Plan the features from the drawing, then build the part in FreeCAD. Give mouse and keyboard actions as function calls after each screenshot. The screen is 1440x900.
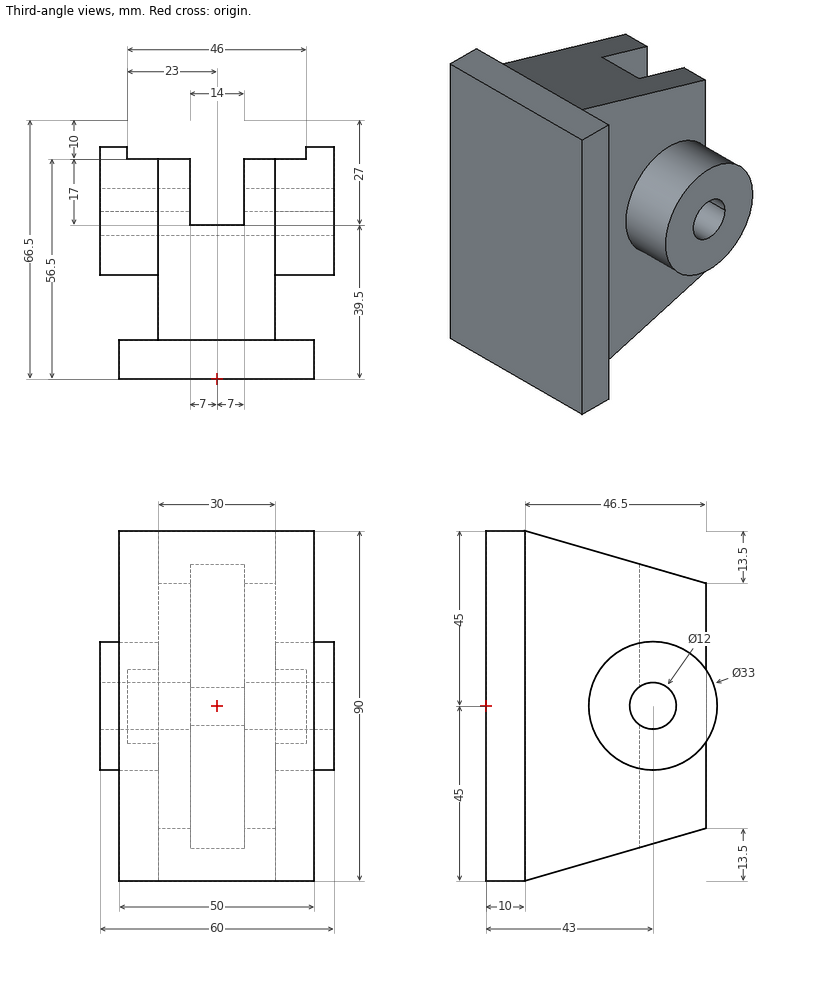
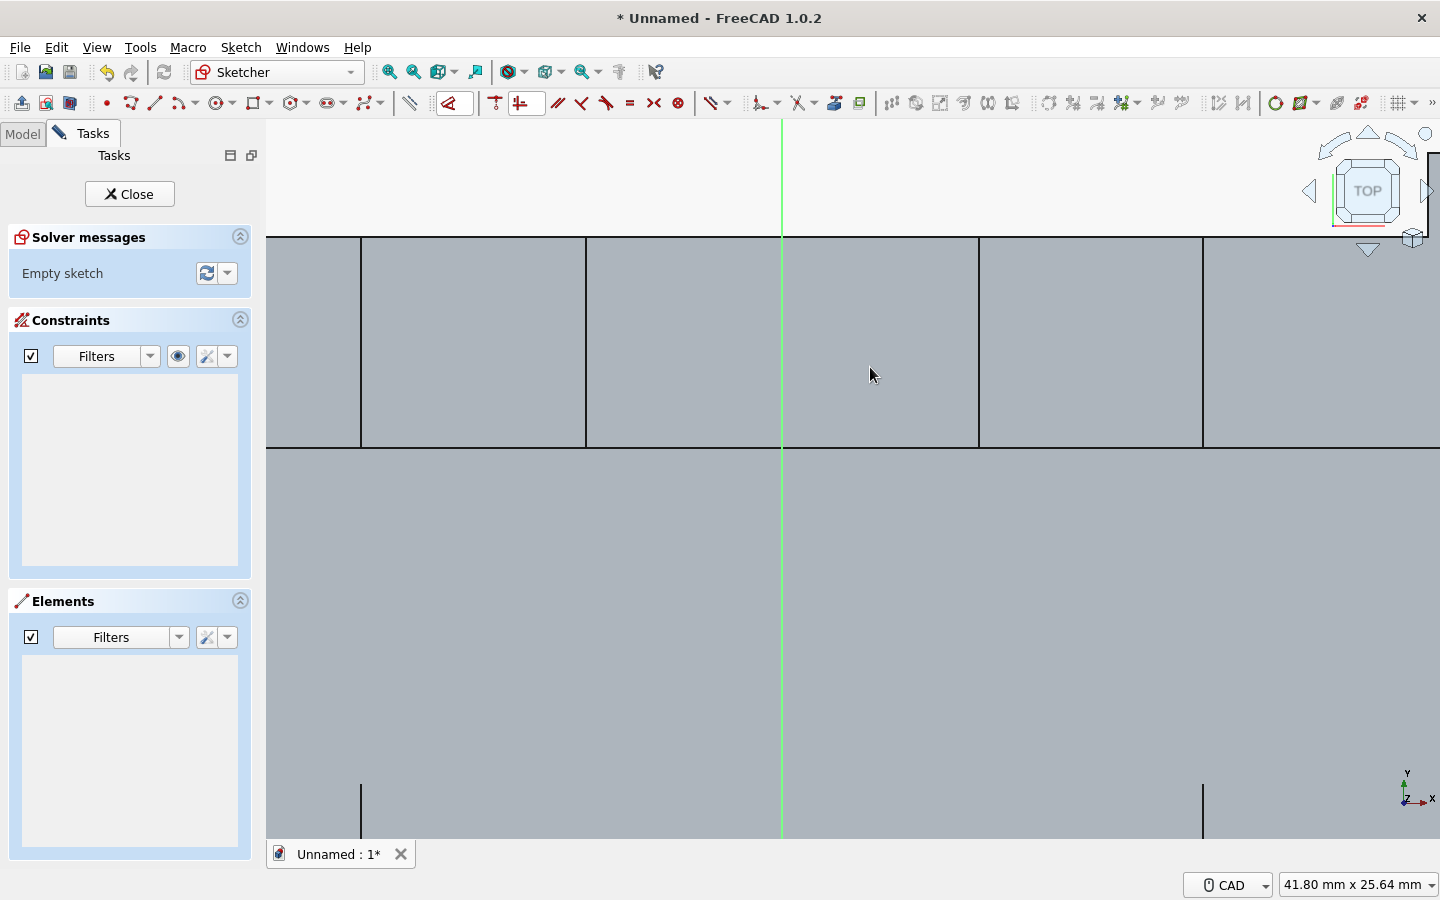
click(254, 104)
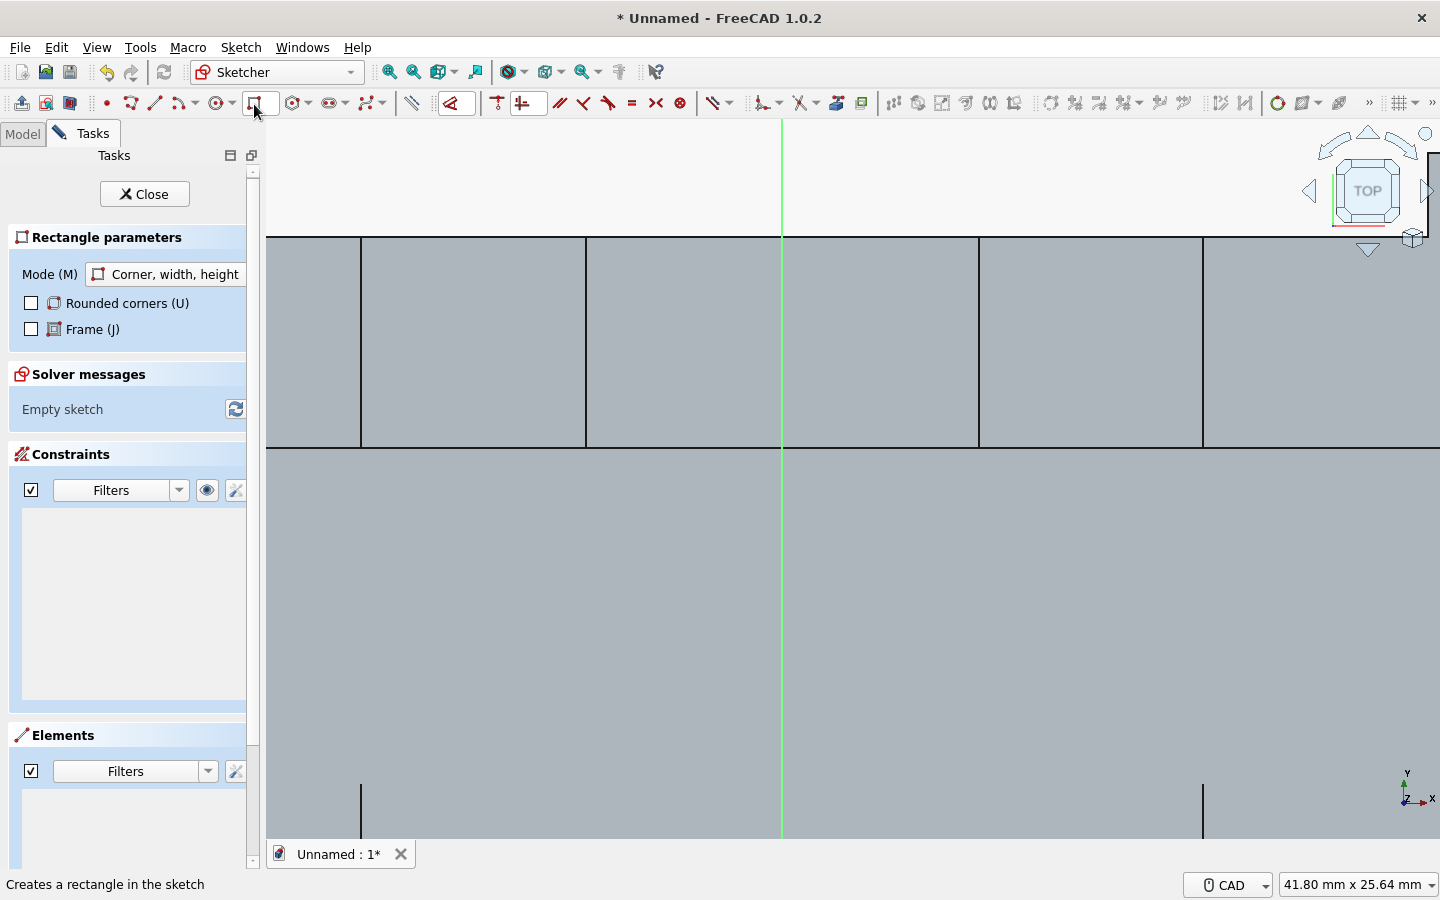
click(586, 237)
click(979, 715)
key(Escape)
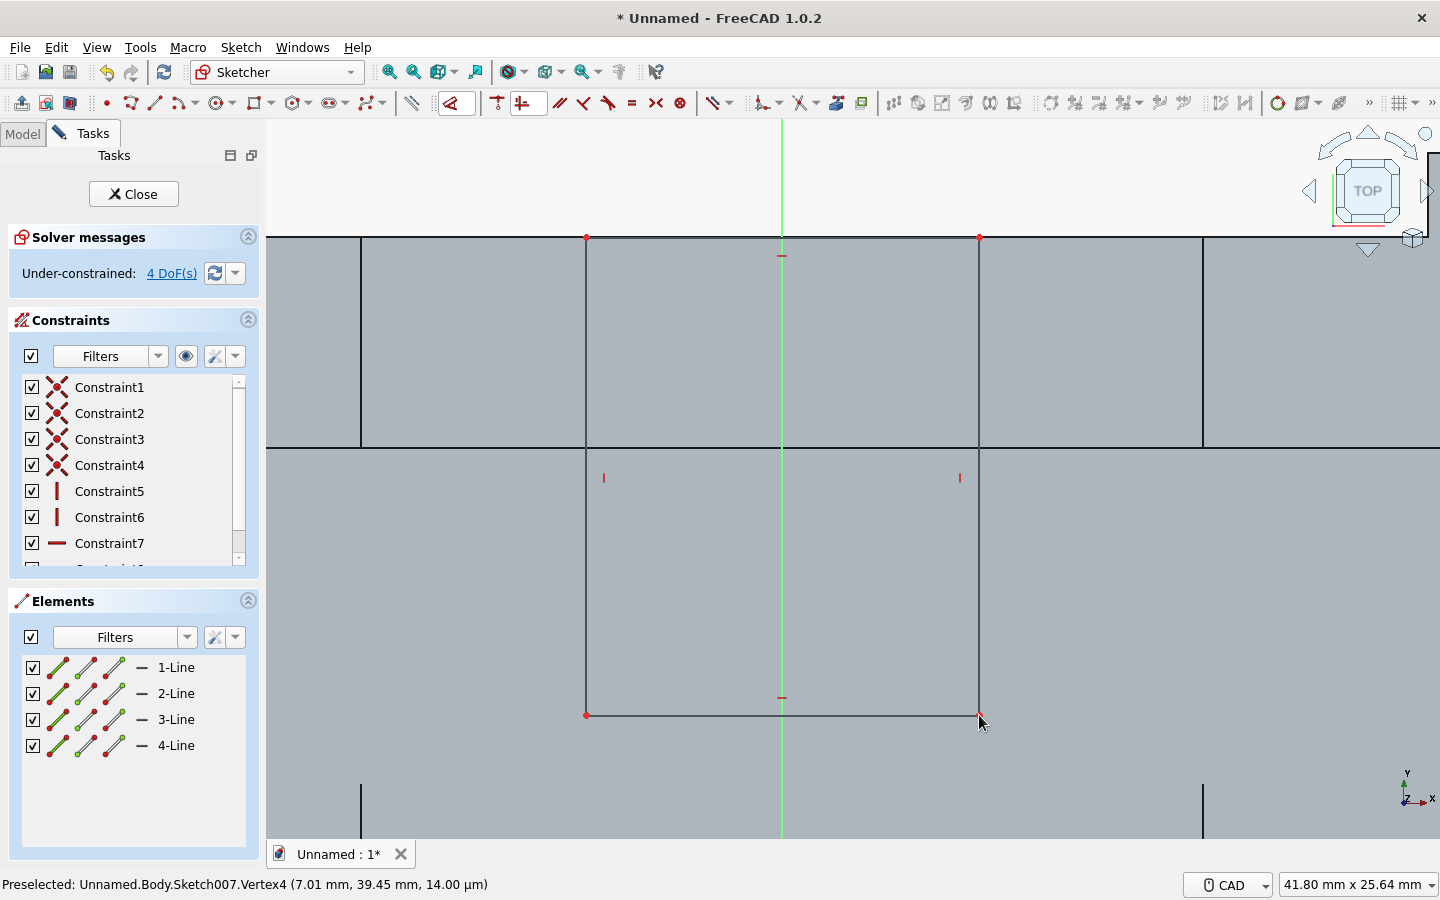
click(586, 381)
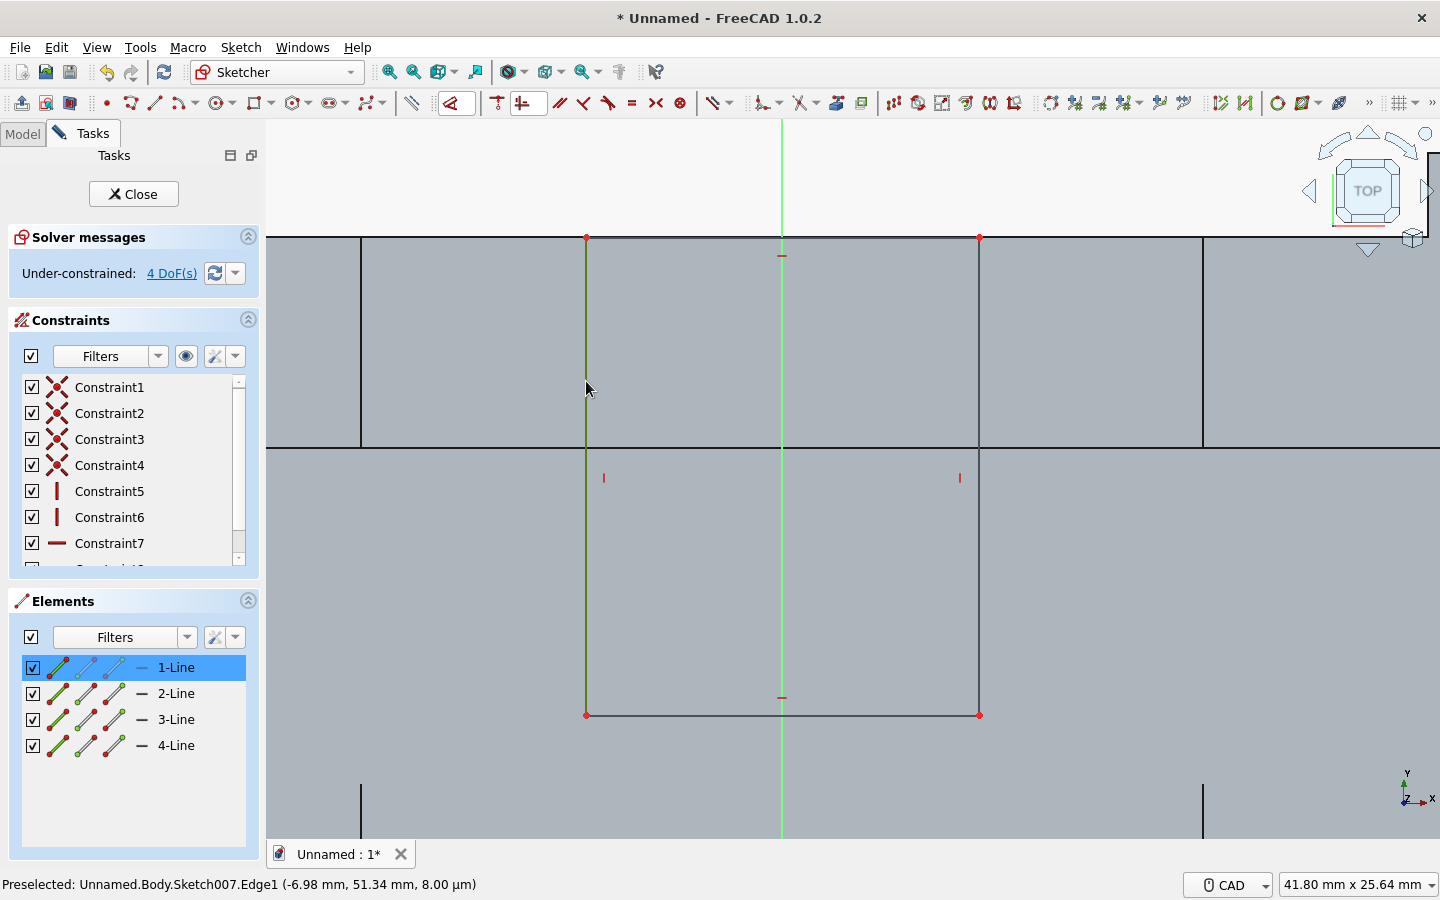
click(470, 104)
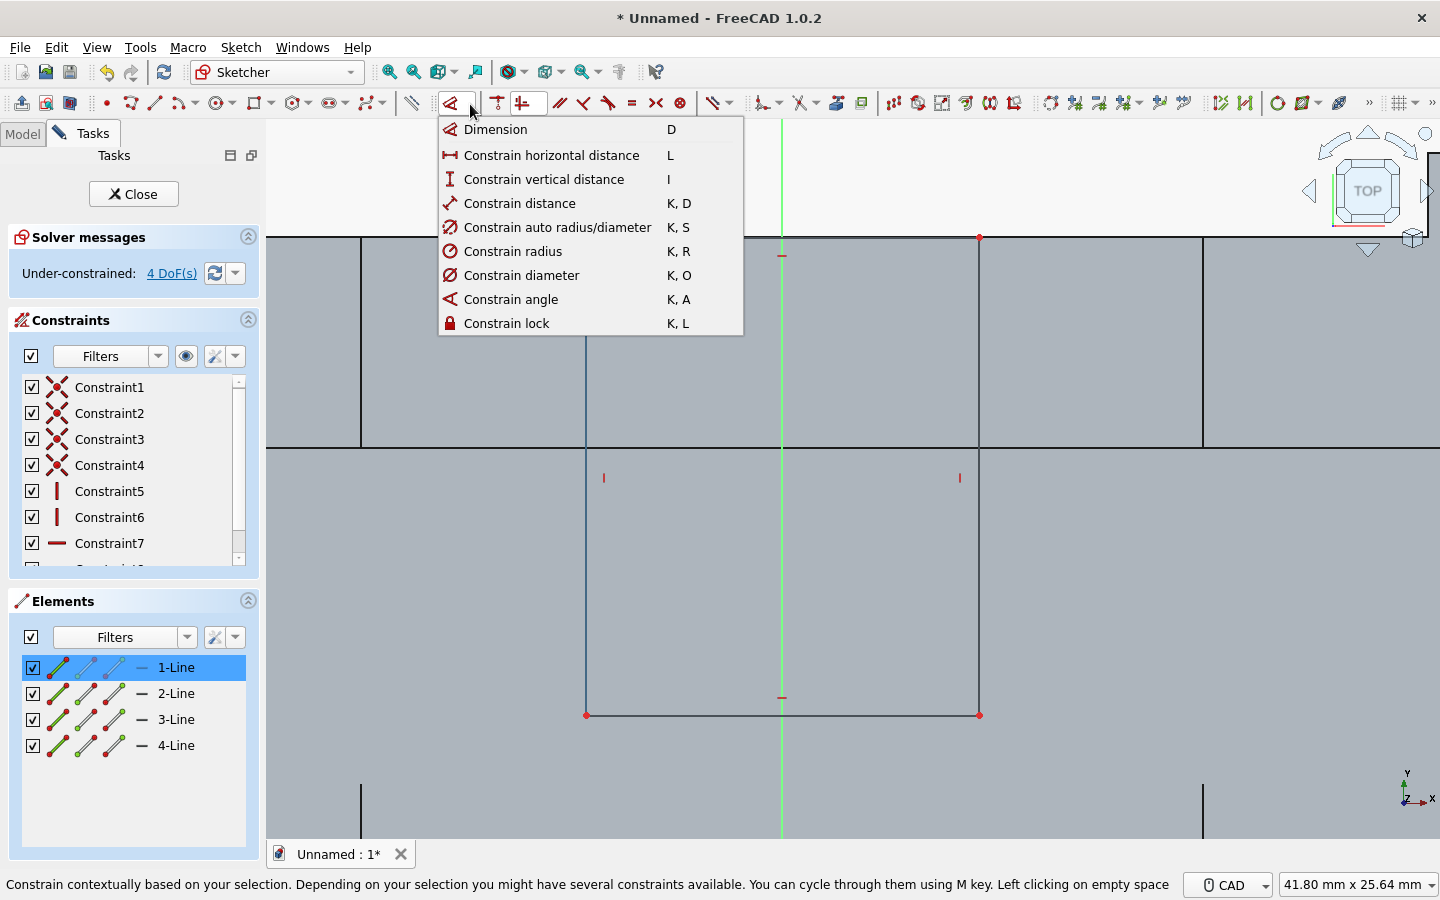
click(591, 179)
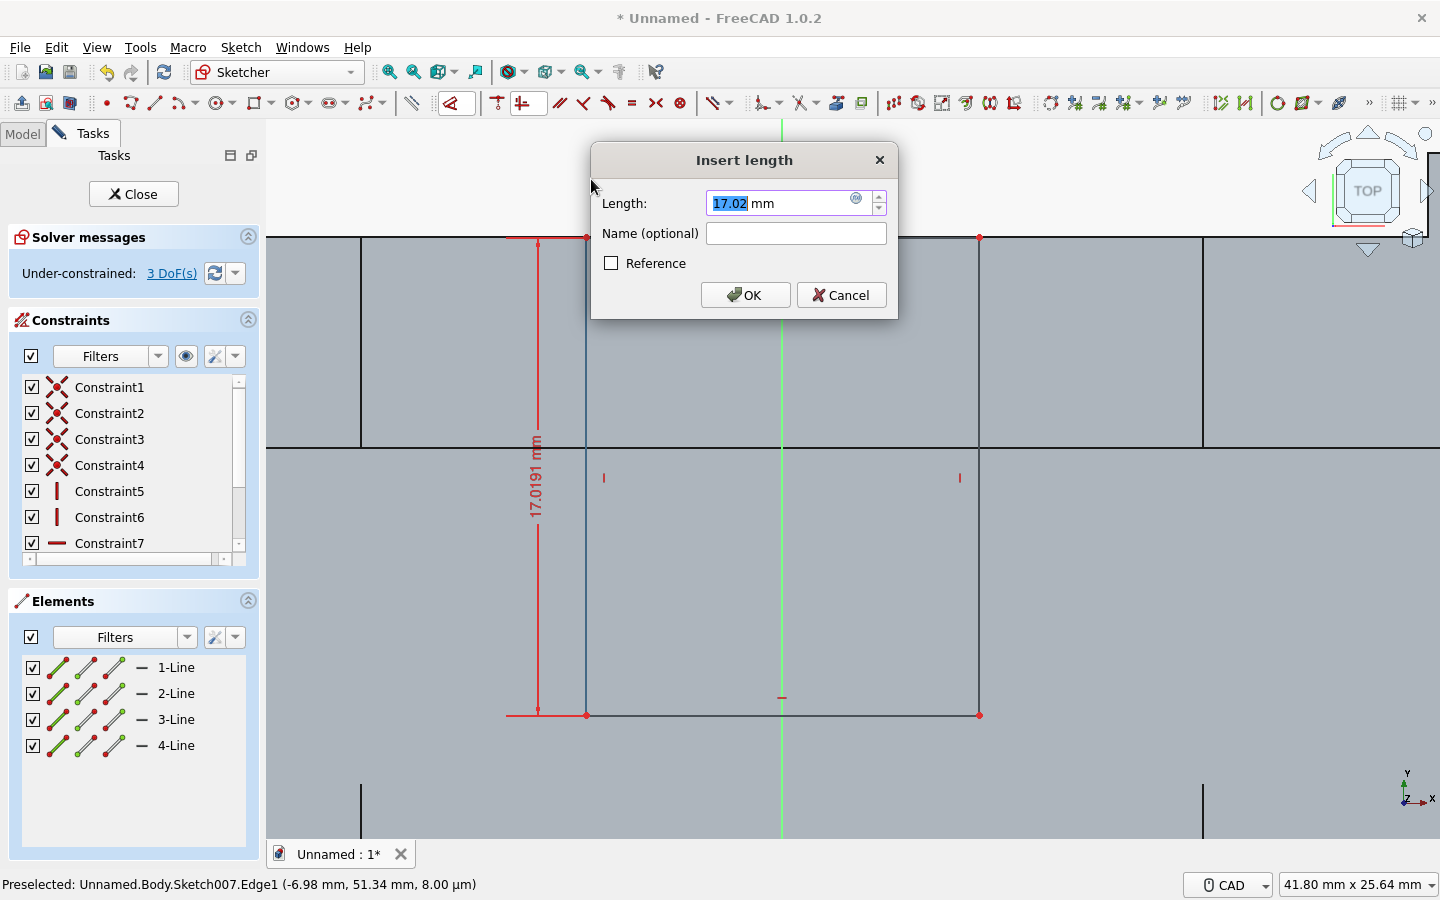
text(17)
key(Return)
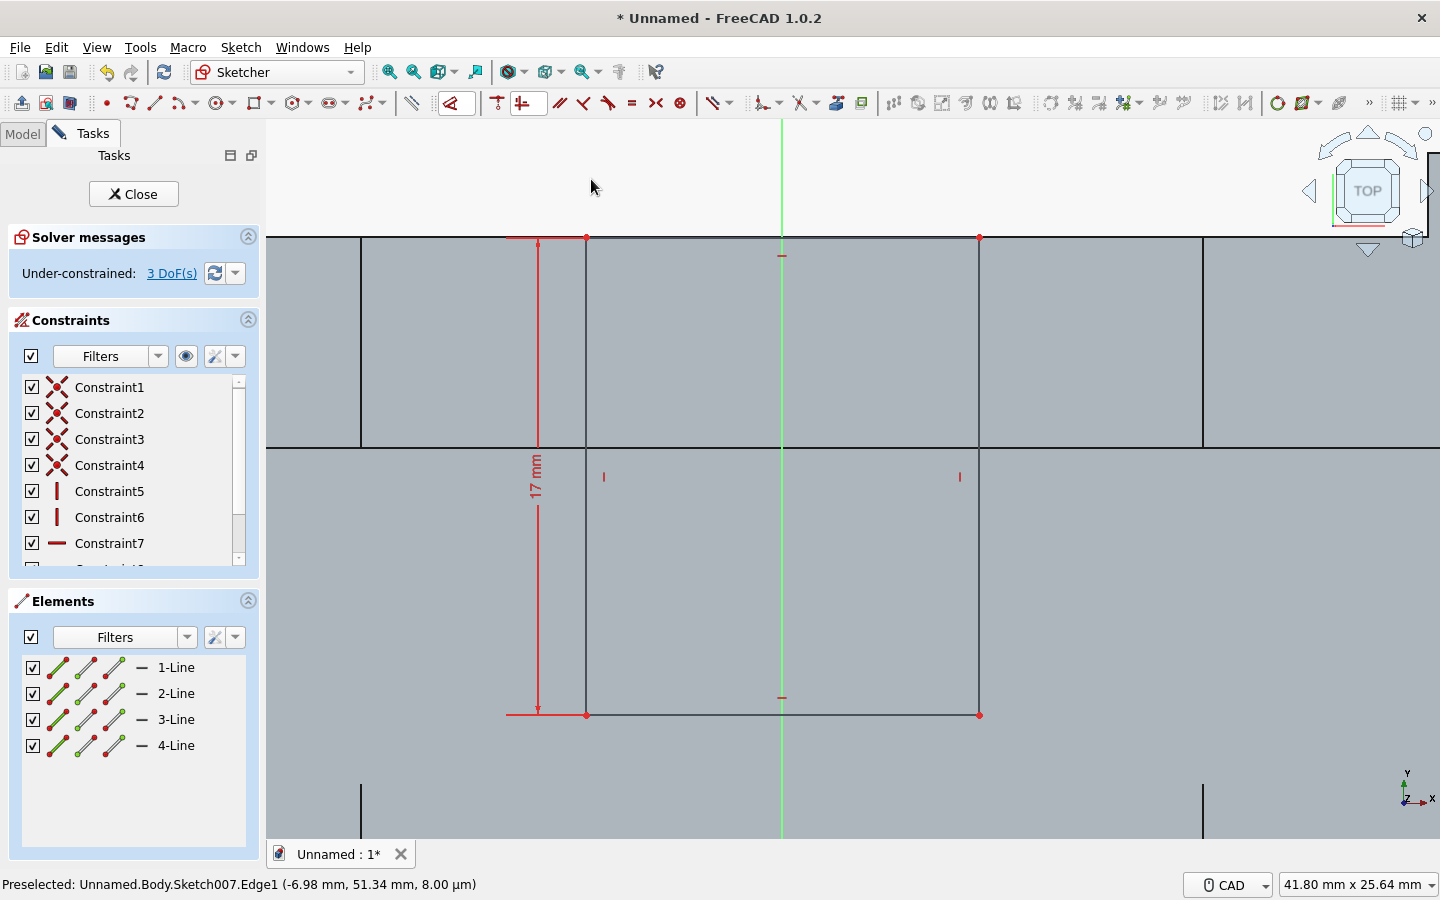
click(704, 715)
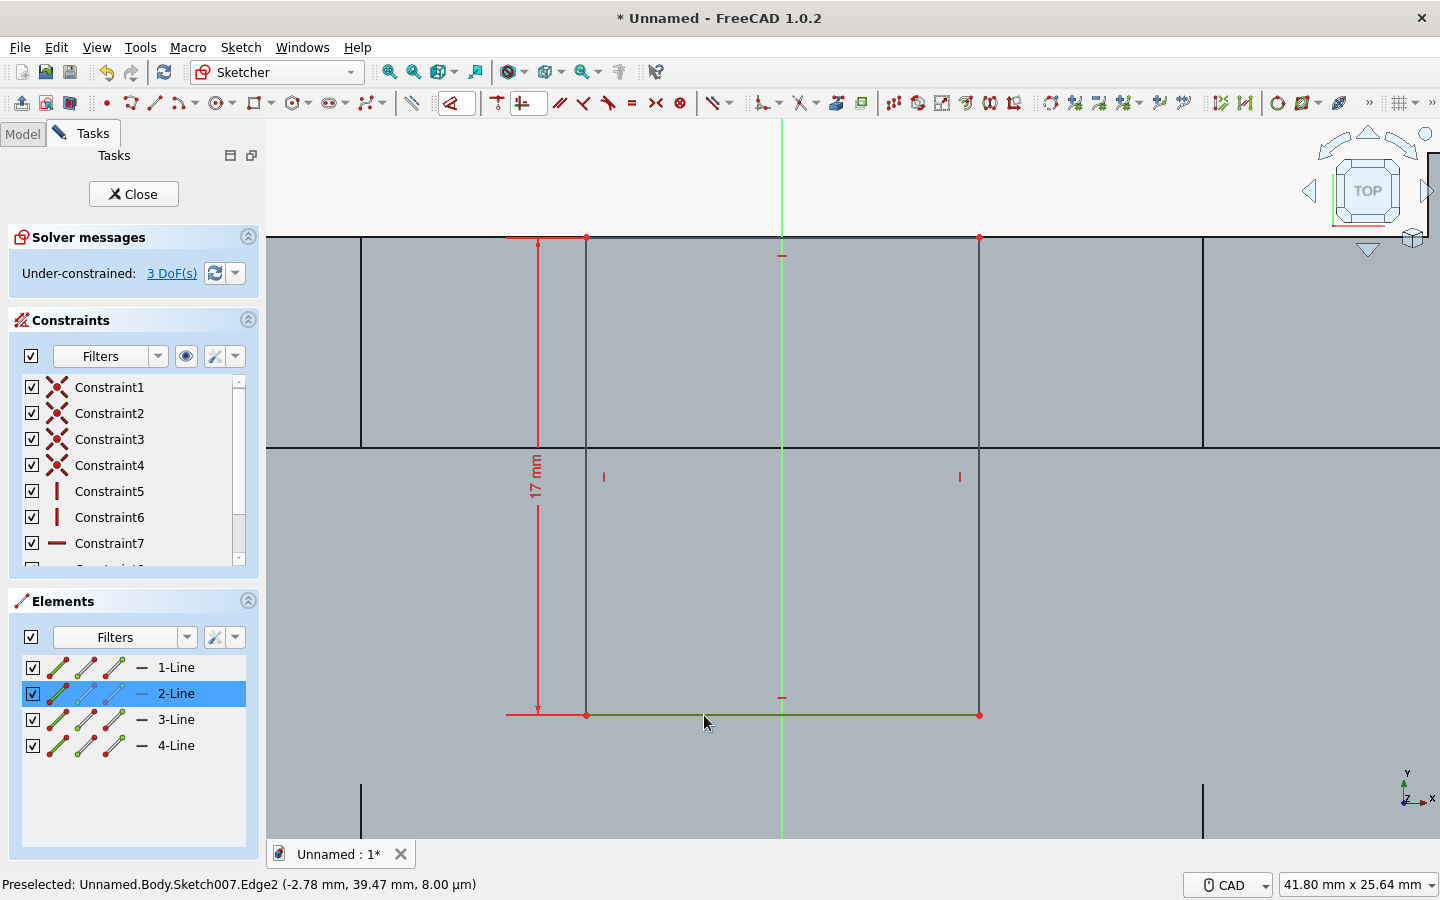
click(470, 104)